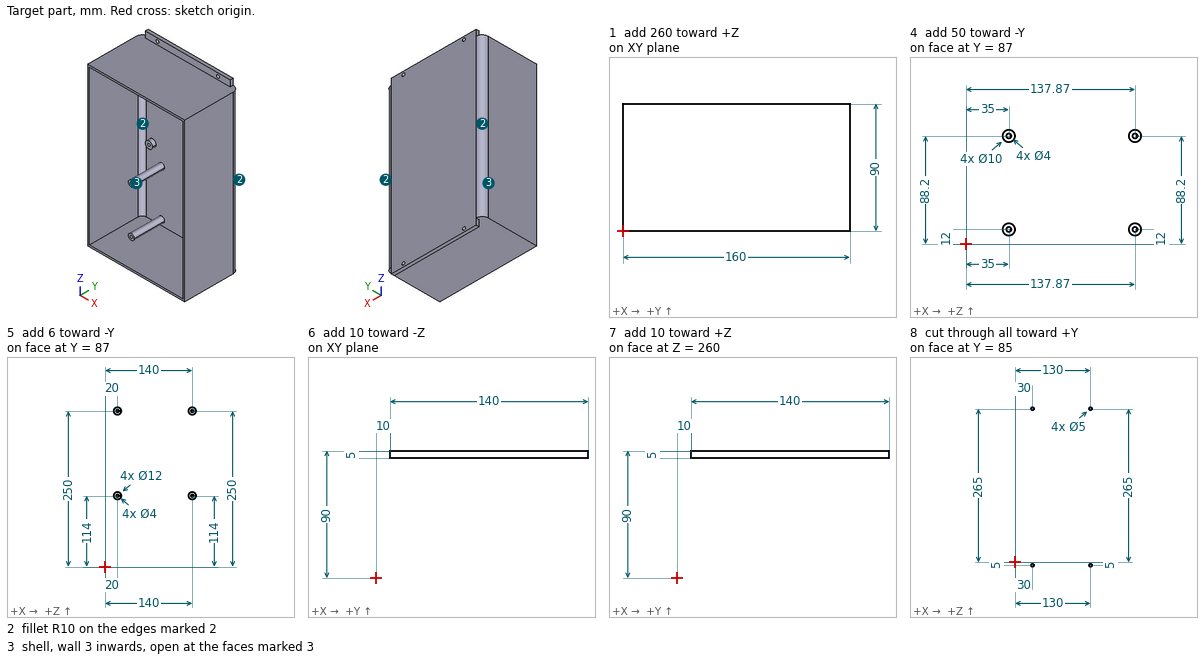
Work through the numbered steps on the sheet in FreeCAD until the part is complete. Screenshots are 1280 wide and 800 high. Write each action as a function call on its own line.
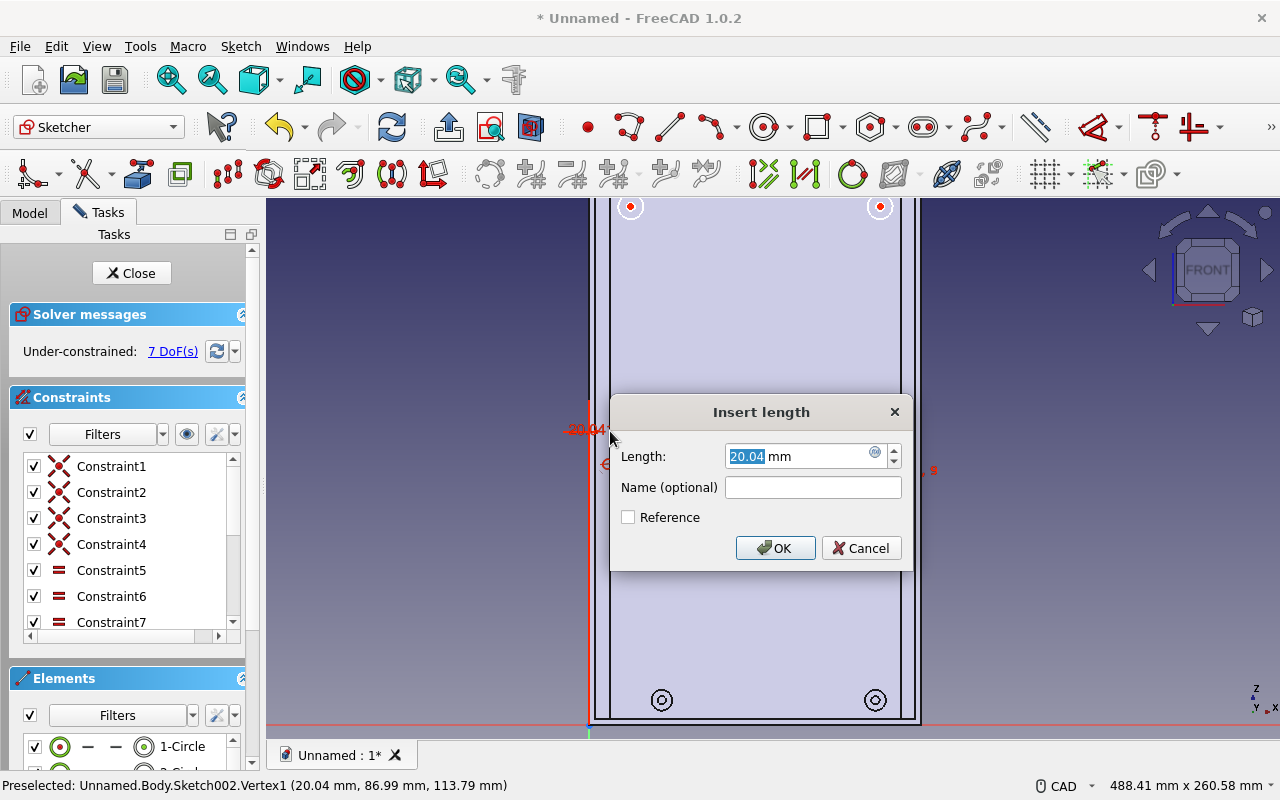
text(20)
key(Return)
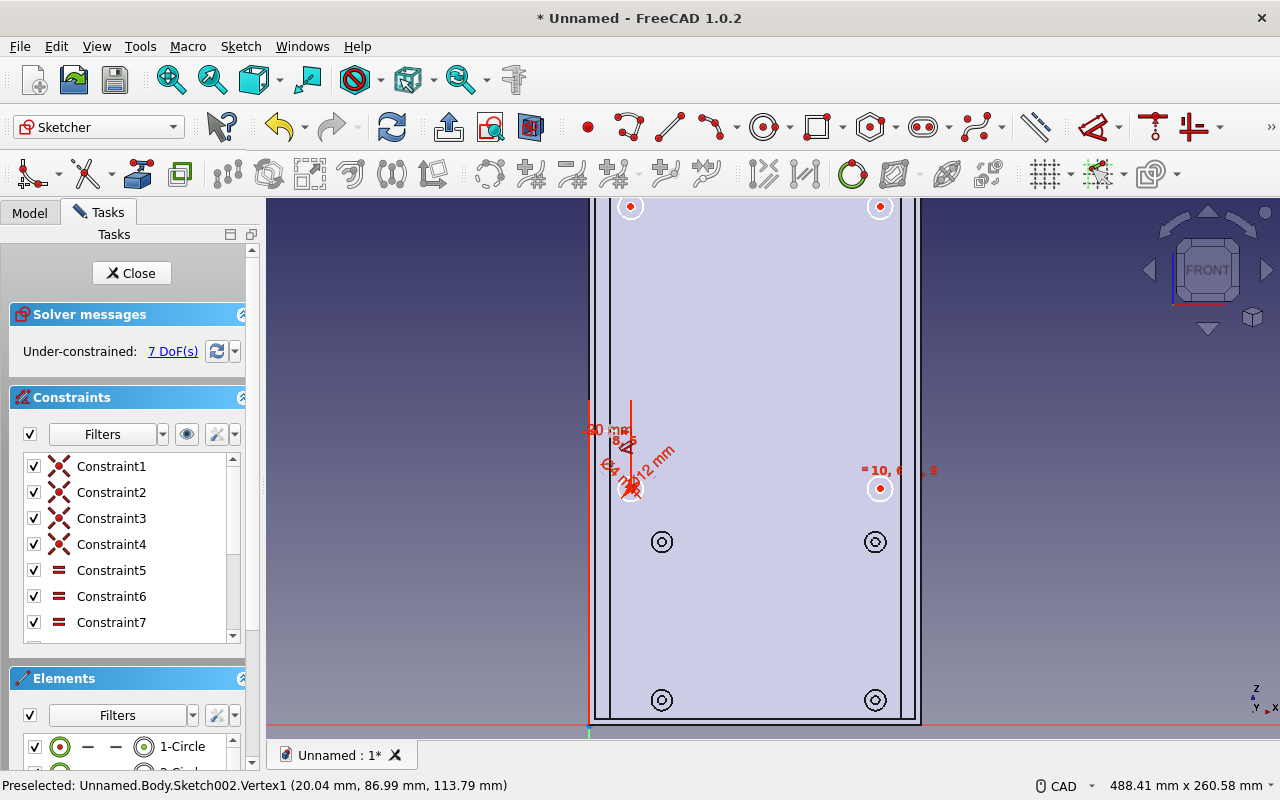
scroll(631, 487, down, 2)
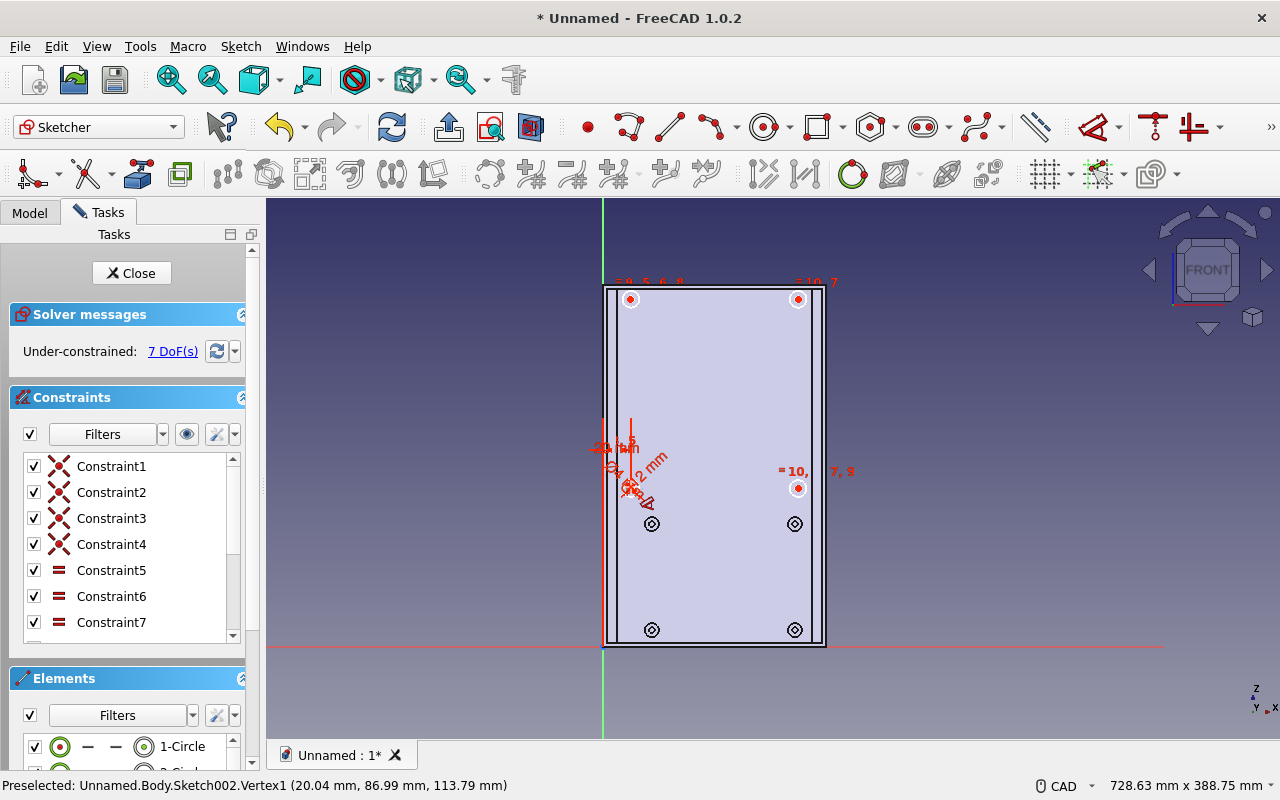
scroll(631, 299, up, 2)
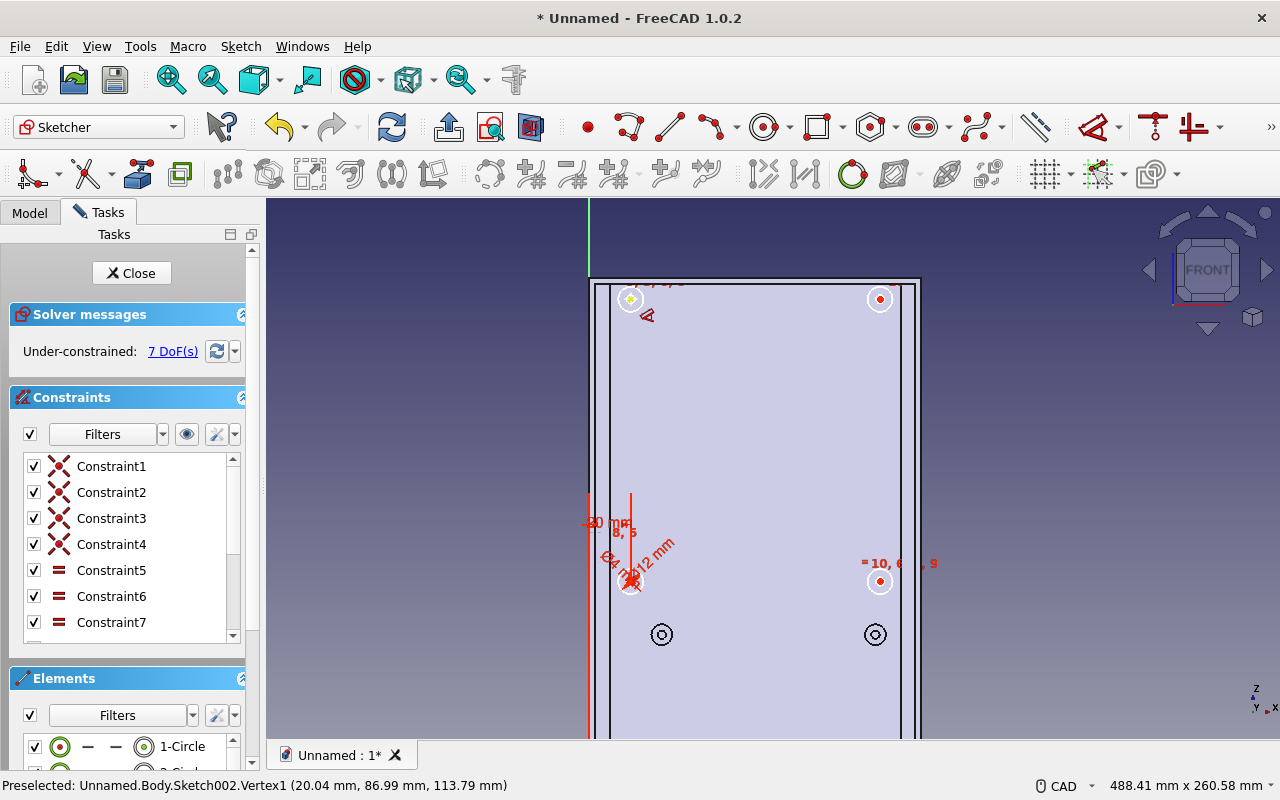
click(631, 299)
click(610, 265)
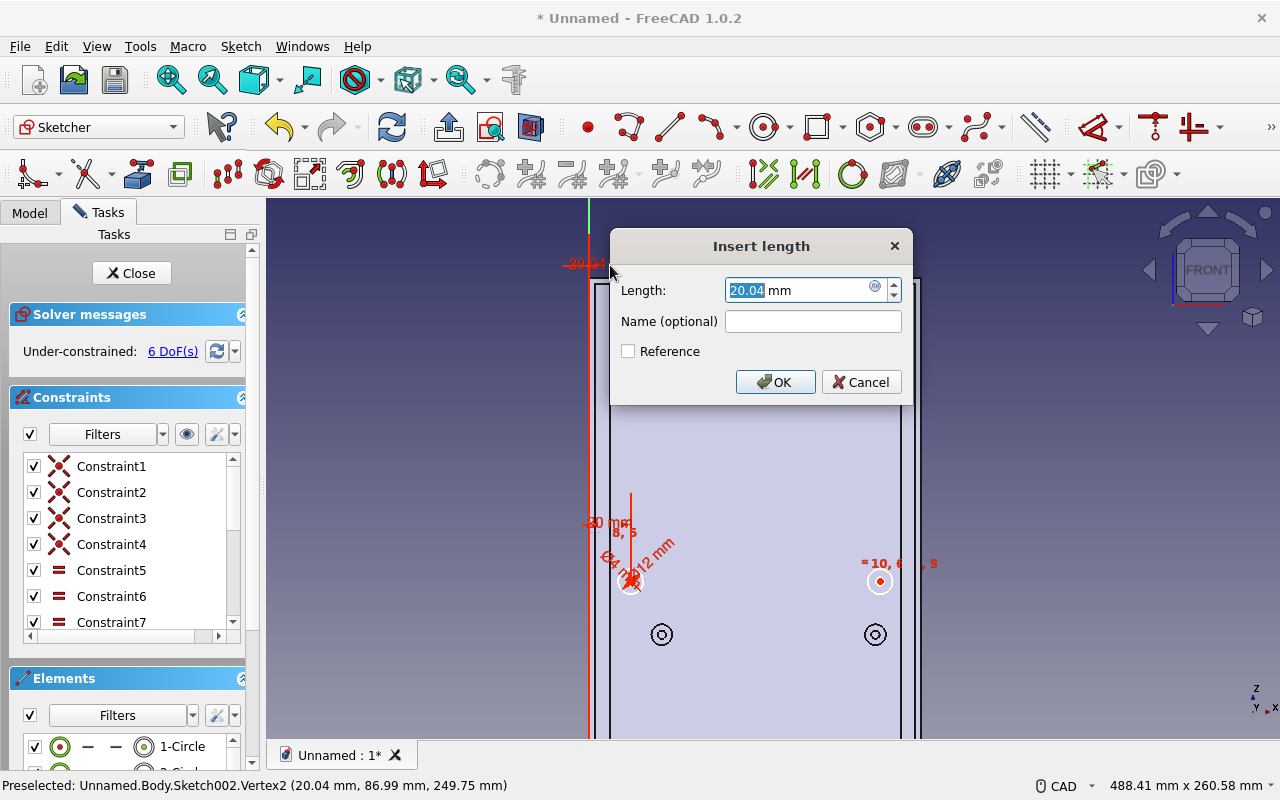
text(20)
key(Return)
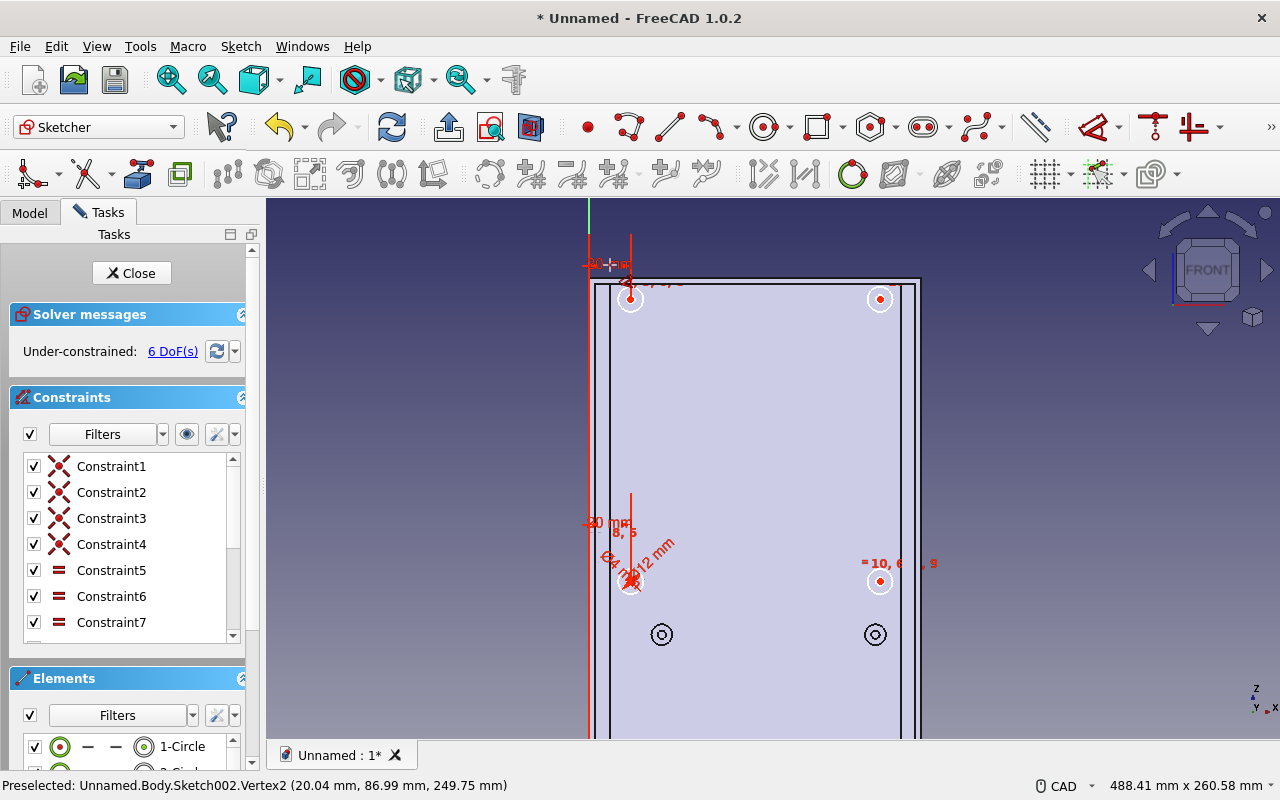
click(631, 582)
click(555, 646)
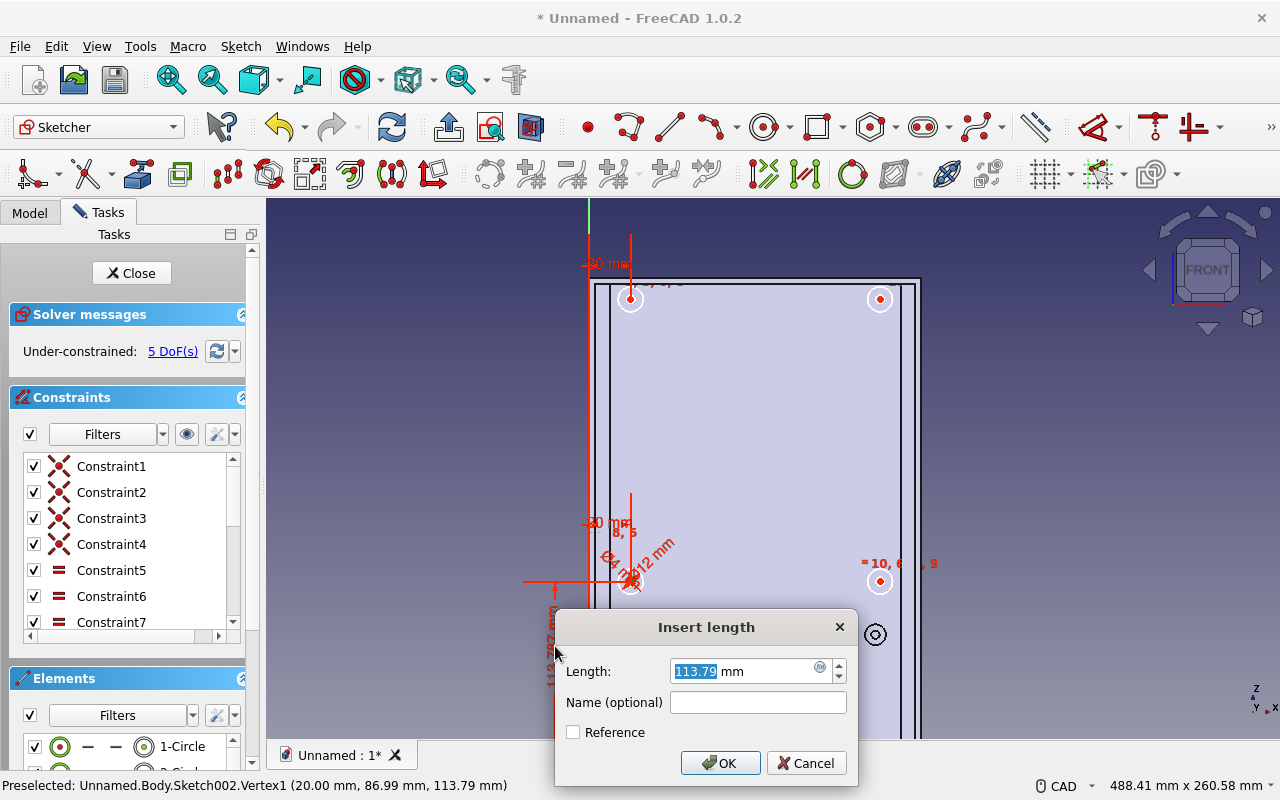
text(114)
key(Return)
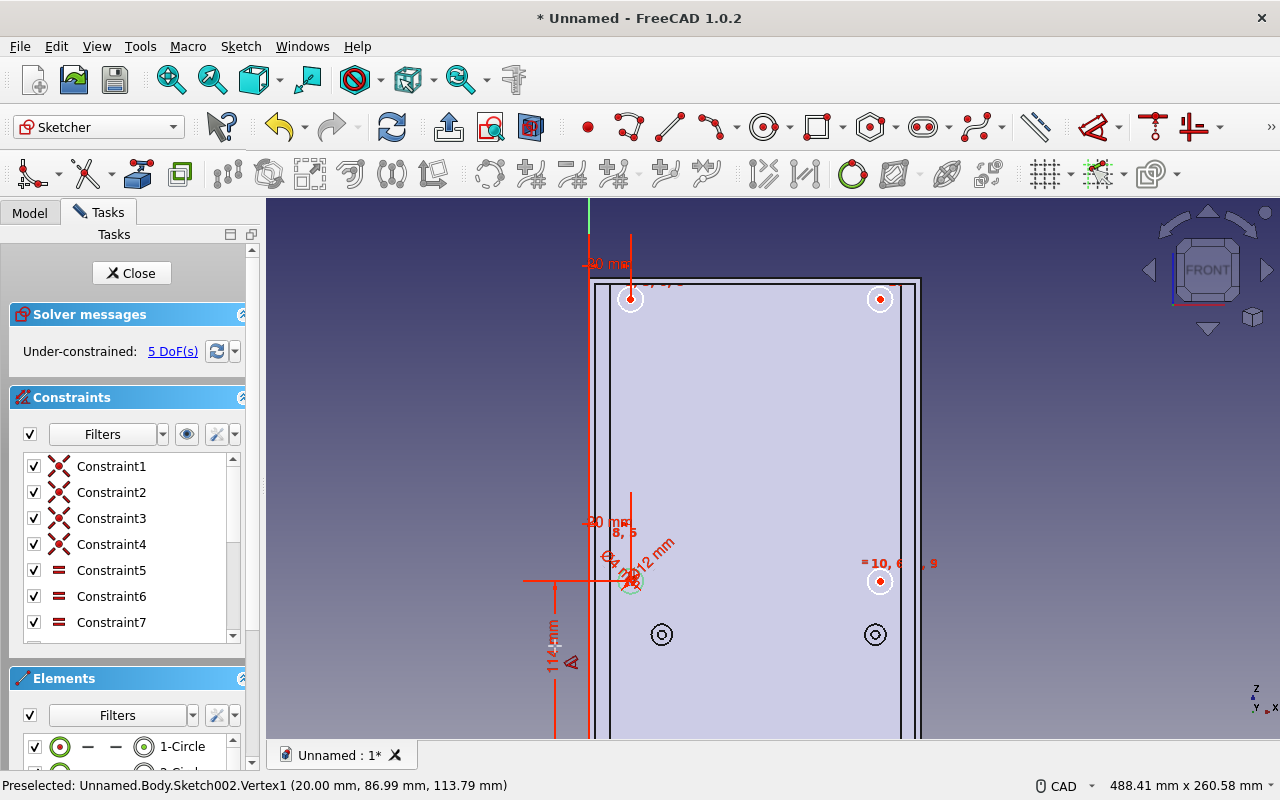
click(631, 299)
click(555, 410)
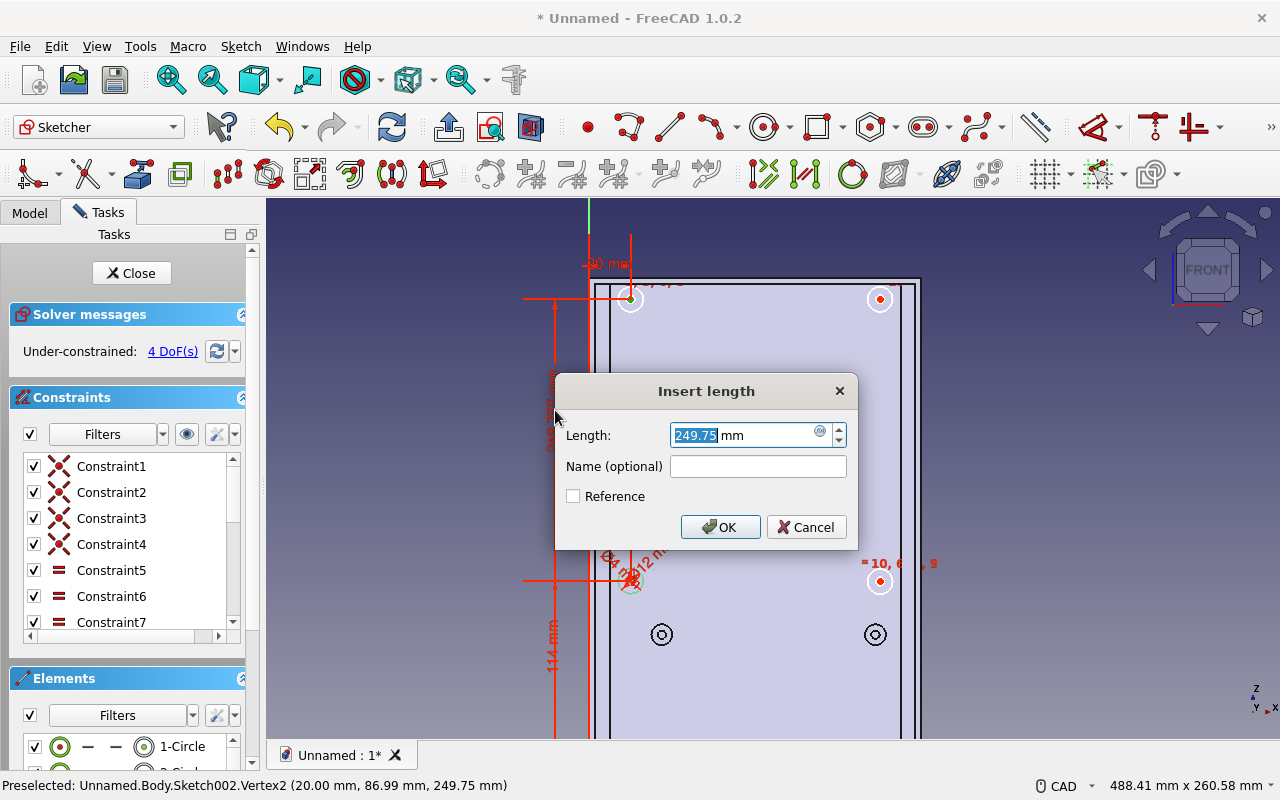
text(250)
key(Return)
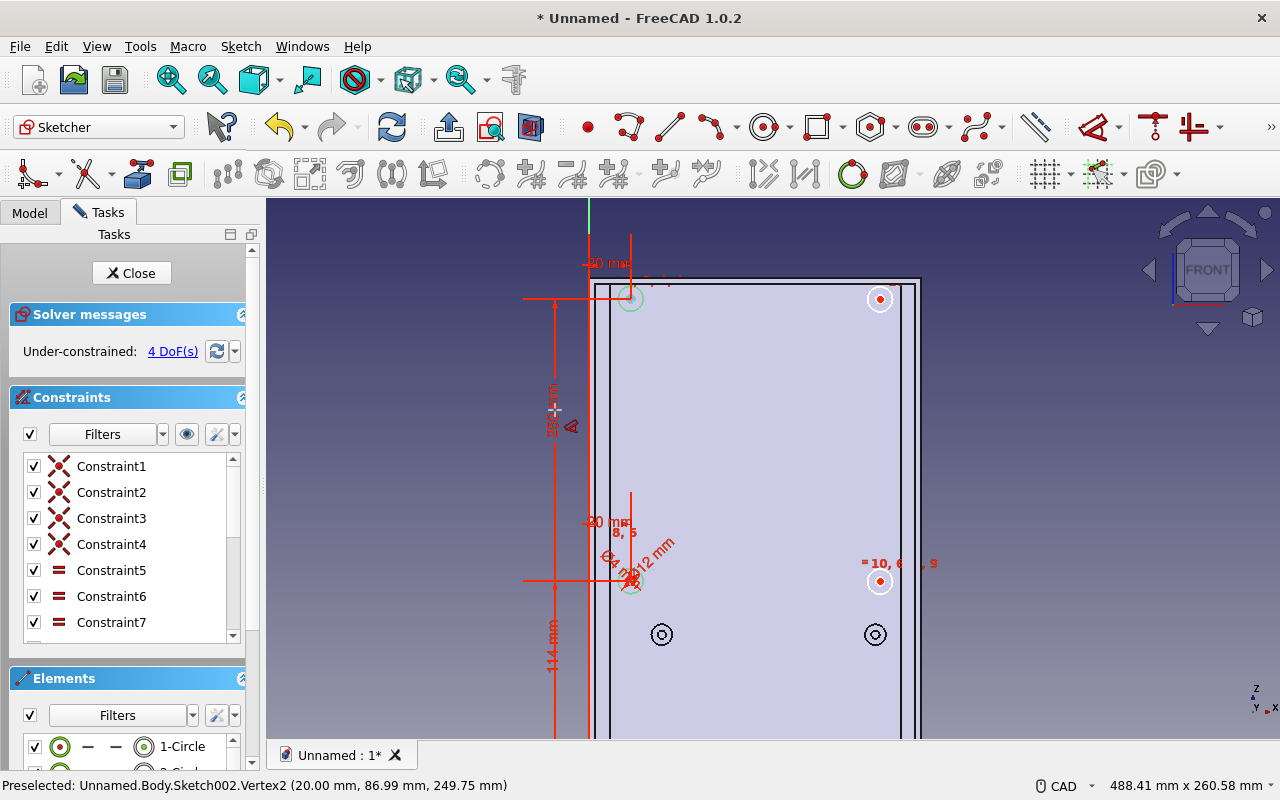
click(880, 582)
click(735, 548)